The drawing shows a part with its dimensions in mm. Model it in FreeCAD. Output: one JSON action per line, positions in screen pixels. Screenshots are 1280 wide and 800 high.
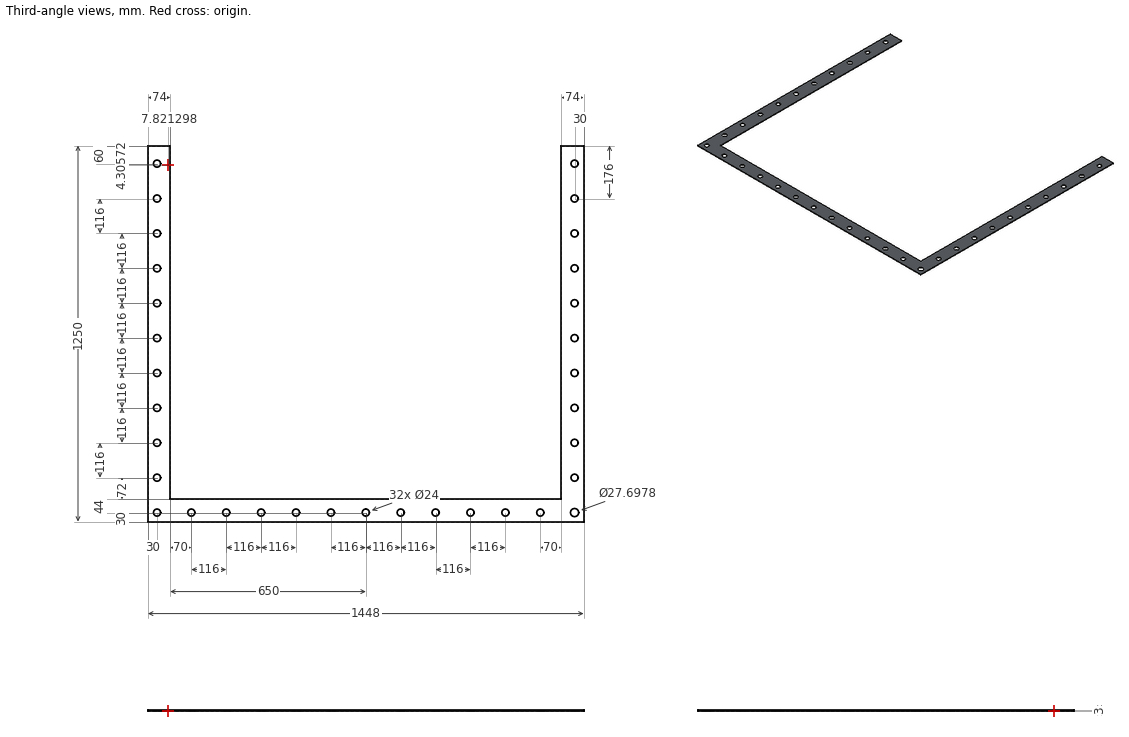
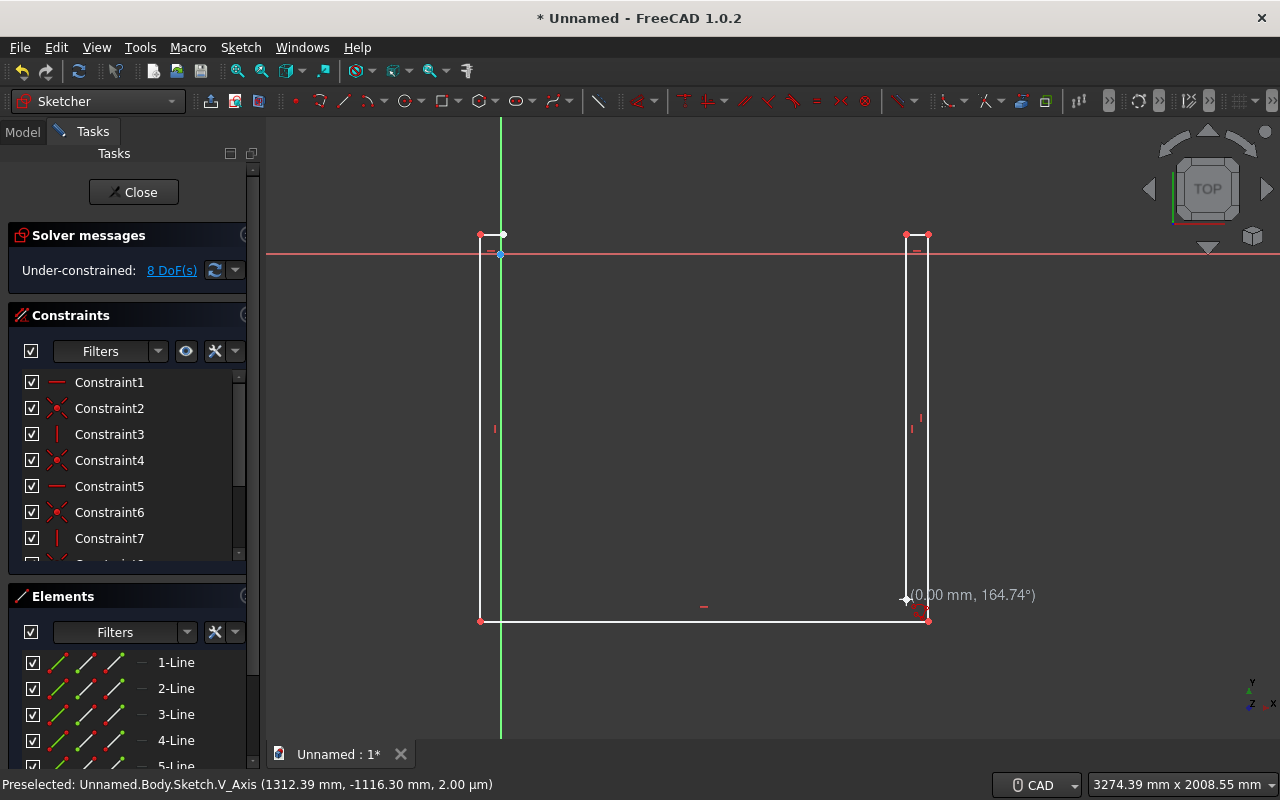
{"action": "scroll", "coordinate": [503, 599], "scroll_direction": "up", "scroll_amount": 10}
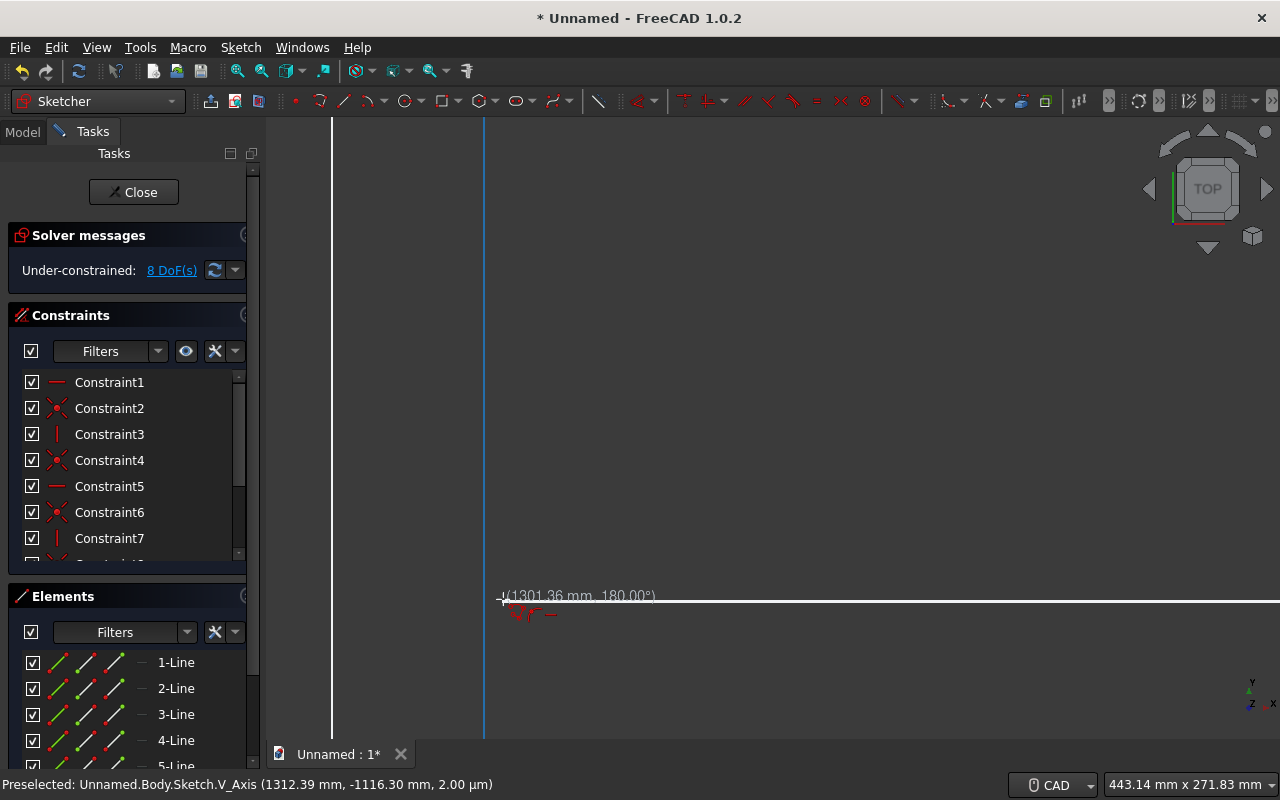
{"action": "left_click", "coordinate": [502, 594]}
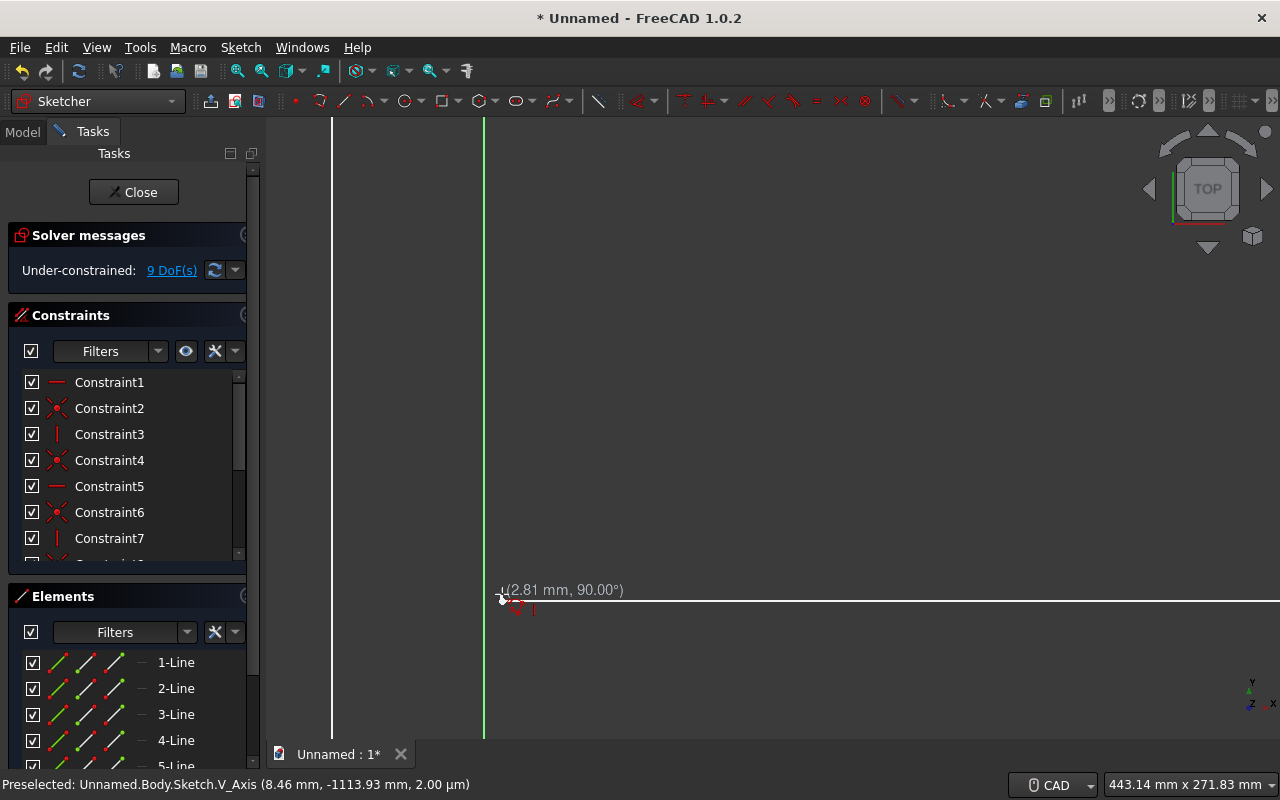
{"action": "scroll", "coordinate": [503, 600], "scroll_direction": "down", "scroll_amount": 10}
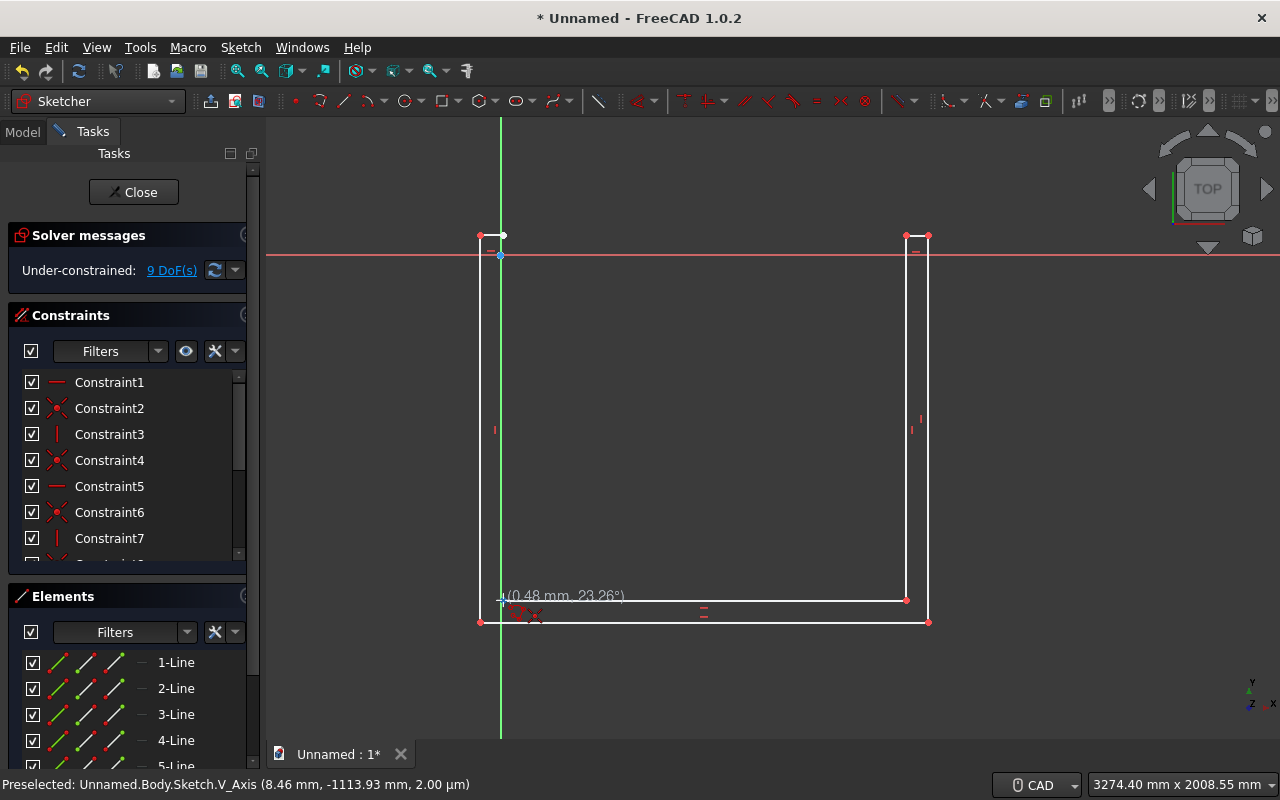
{"action": "scroll", "coordinate": [503, 235], "scroll_direction": "up", "scroll_amount": 10}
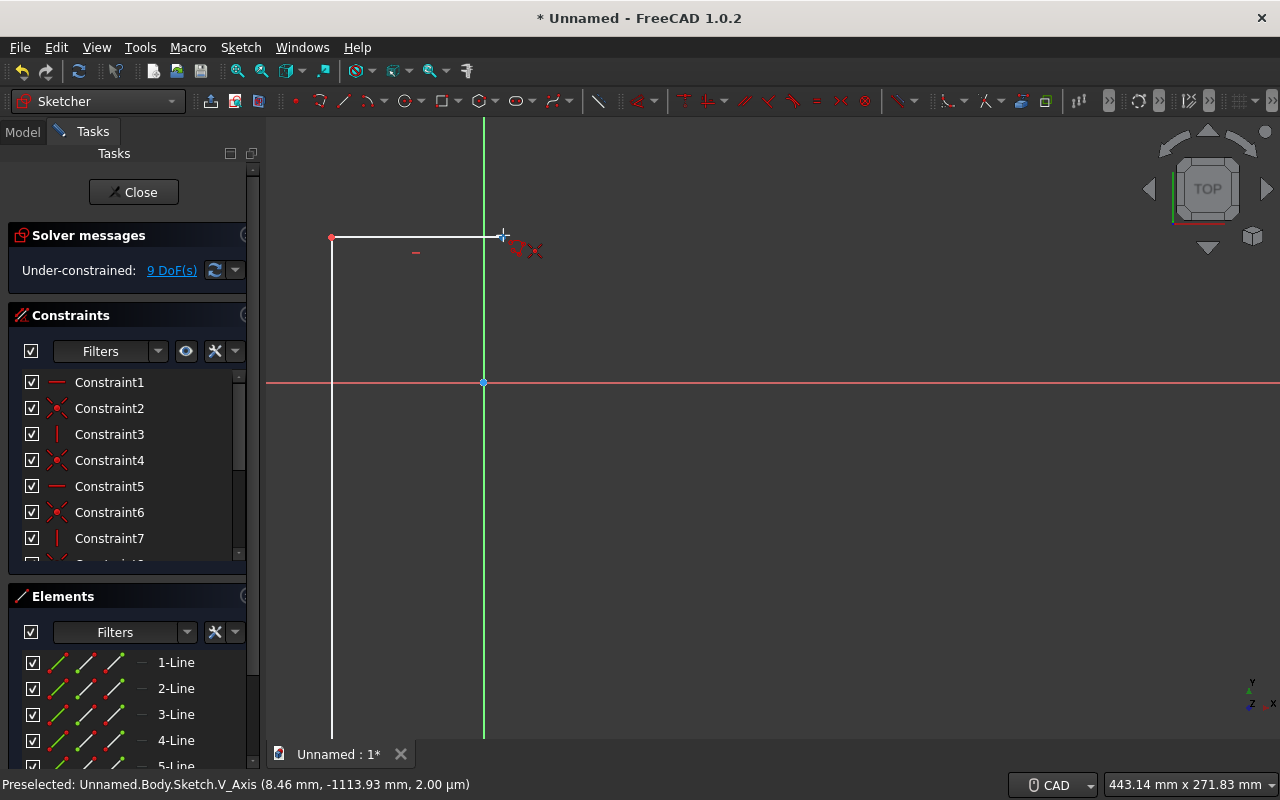
{"action": "left_click", "coordinate": [502, 237]}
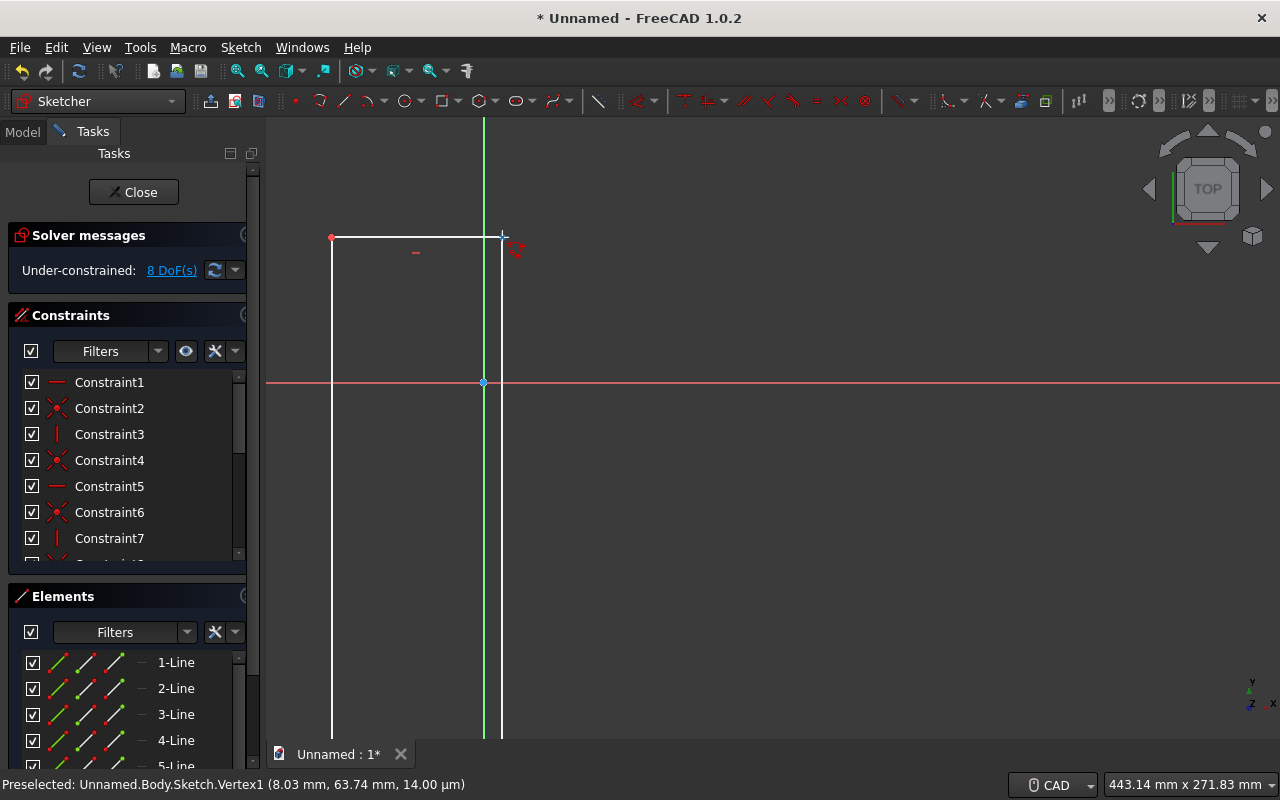
{"action": "left_click", "coordinate": [406, 102]}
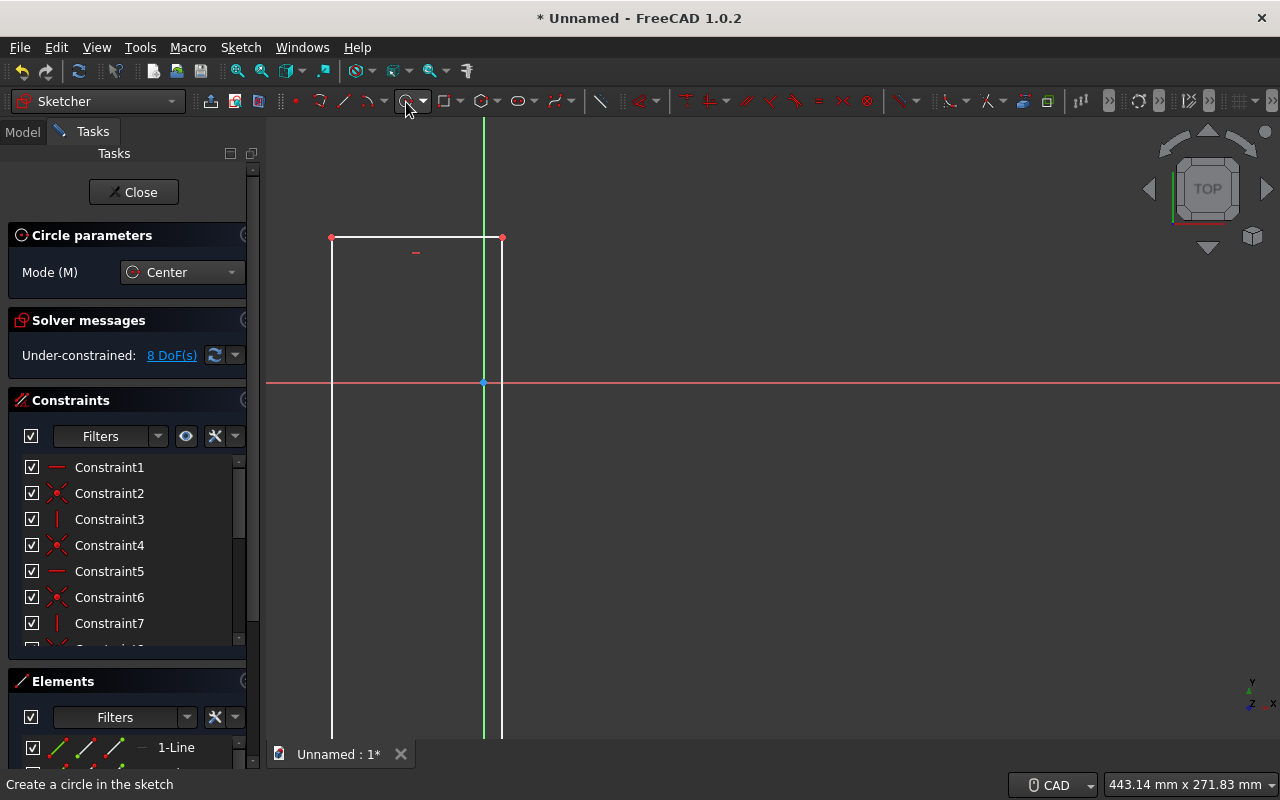
{"action": "scroll", "coordinate": [503, 234], "scroll_direction": "down", "scroll_amount": 10}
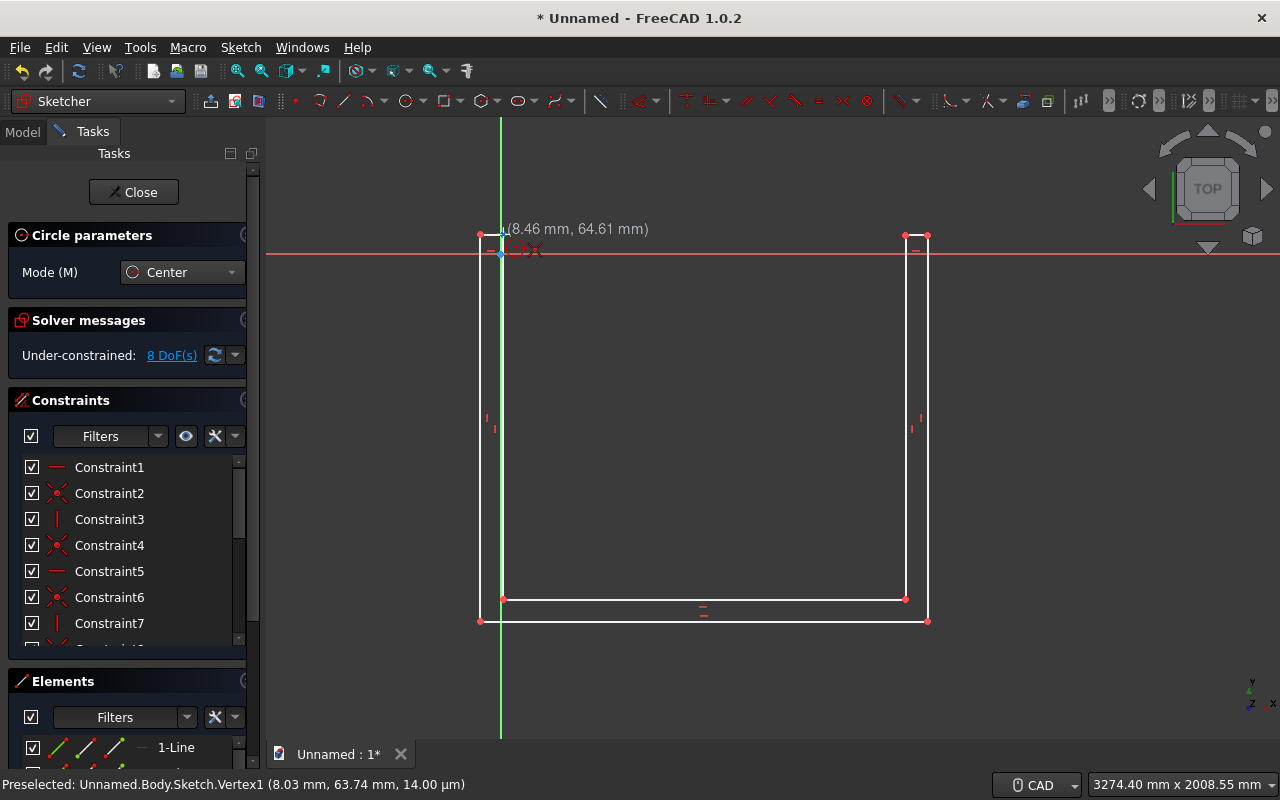
{"action": "scroll", "coordinate": [704, 612], "scroll_direction": "up", "scroll_amount": 10}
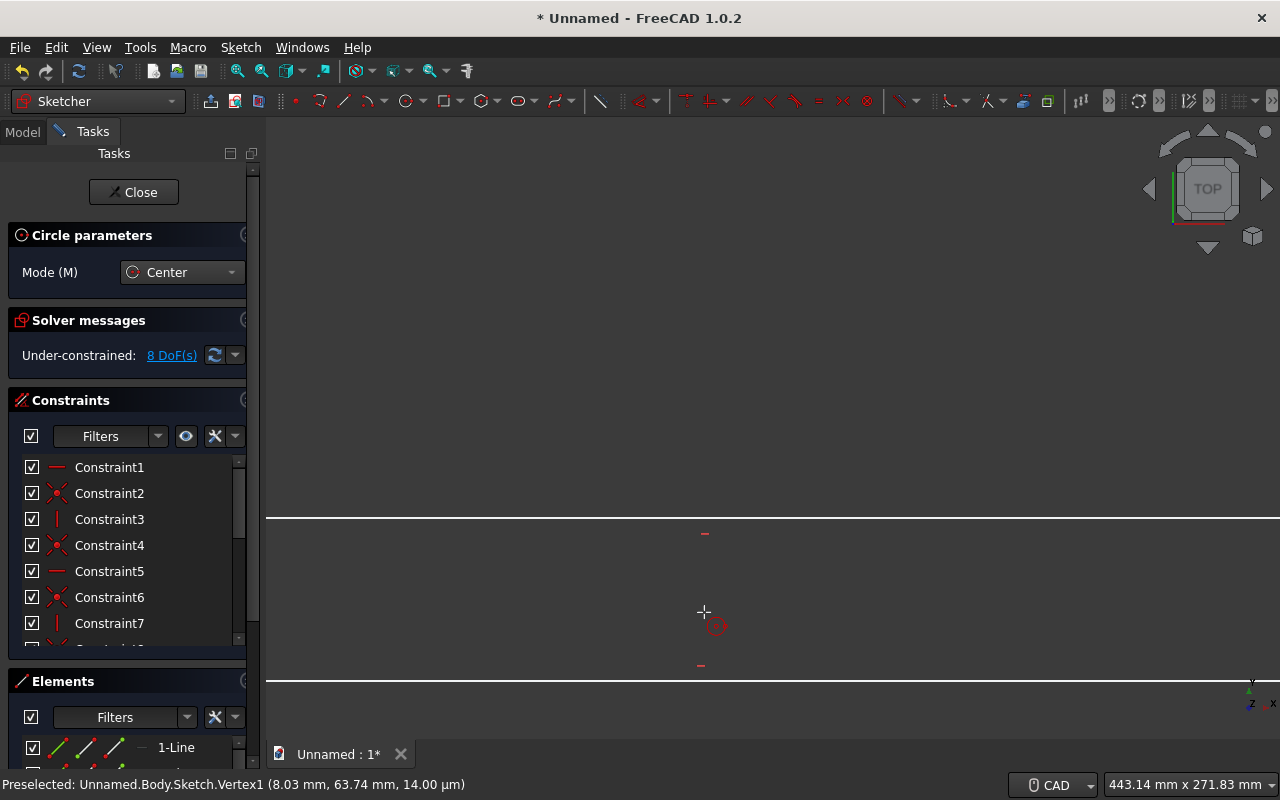
{"action": "scroll", "coordinate": [705, 613], "scroll_direction": "down", "scroll_amount": 10}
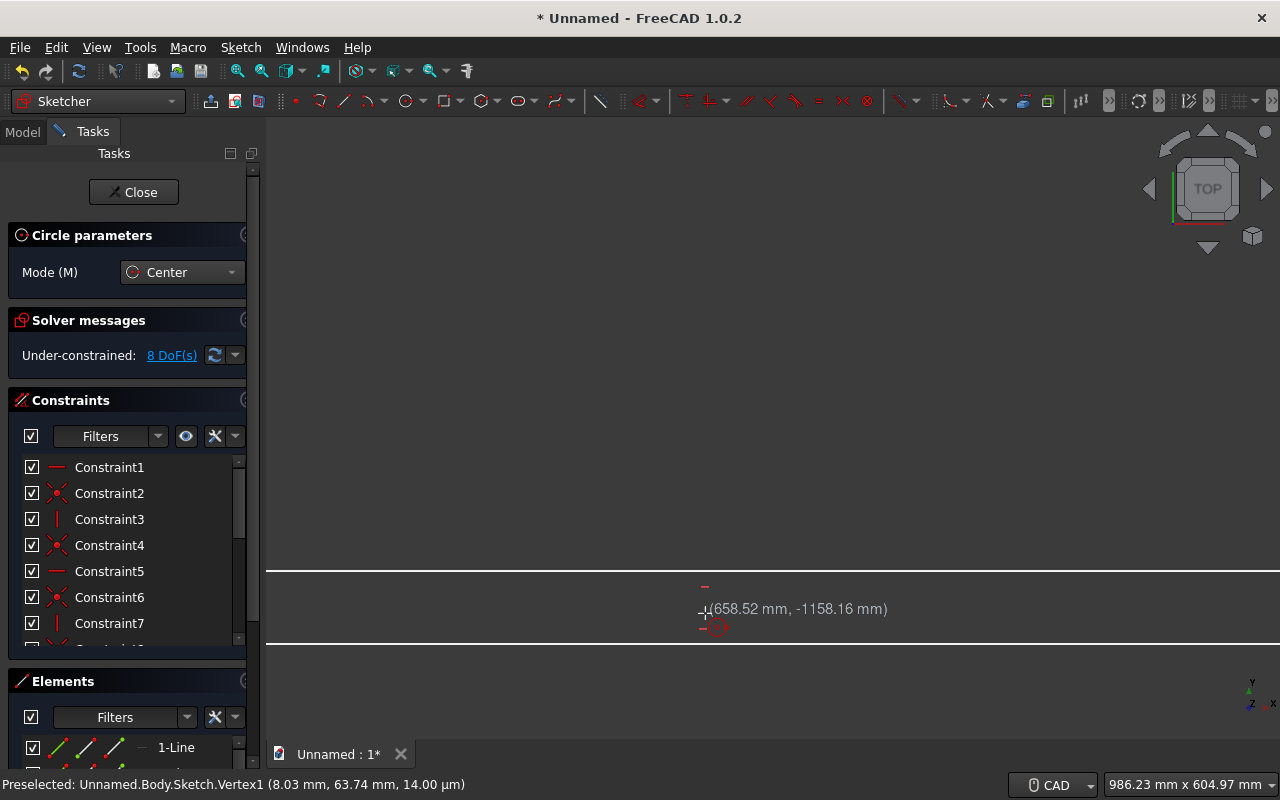
{"action": "scroll", "coordinate": [705, 613], "scroll_direction": "up", "scroll_amount": 3}